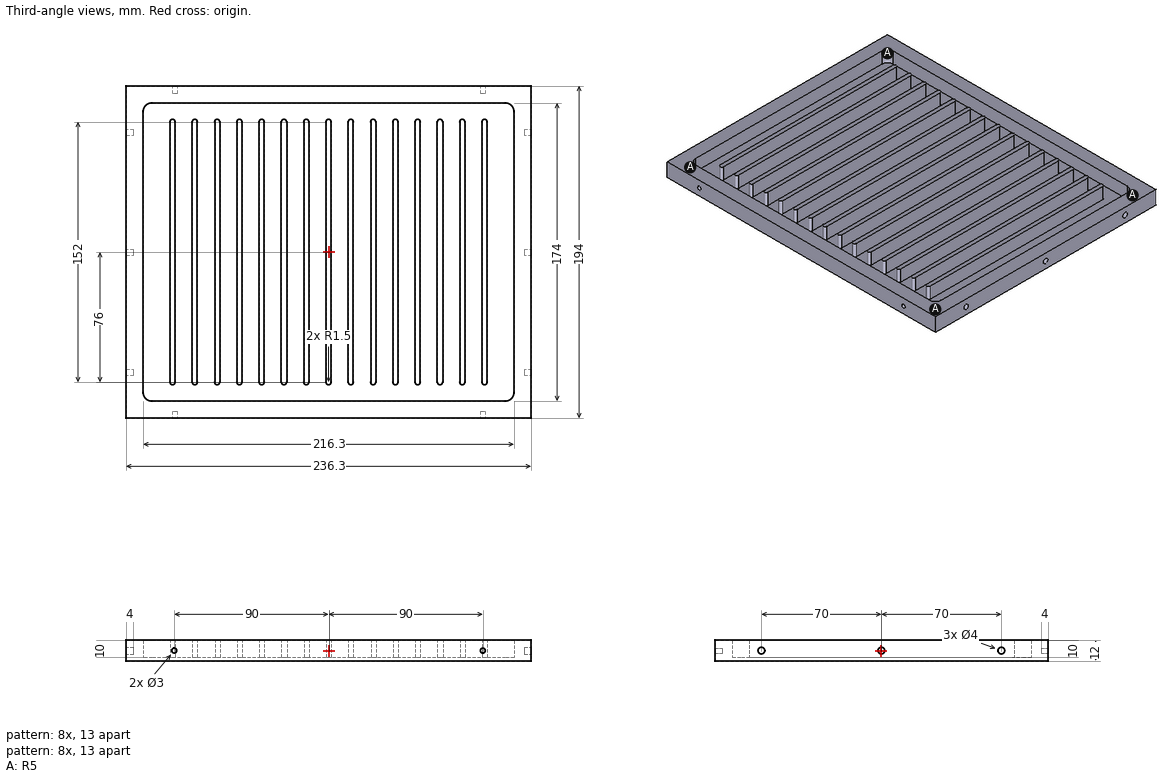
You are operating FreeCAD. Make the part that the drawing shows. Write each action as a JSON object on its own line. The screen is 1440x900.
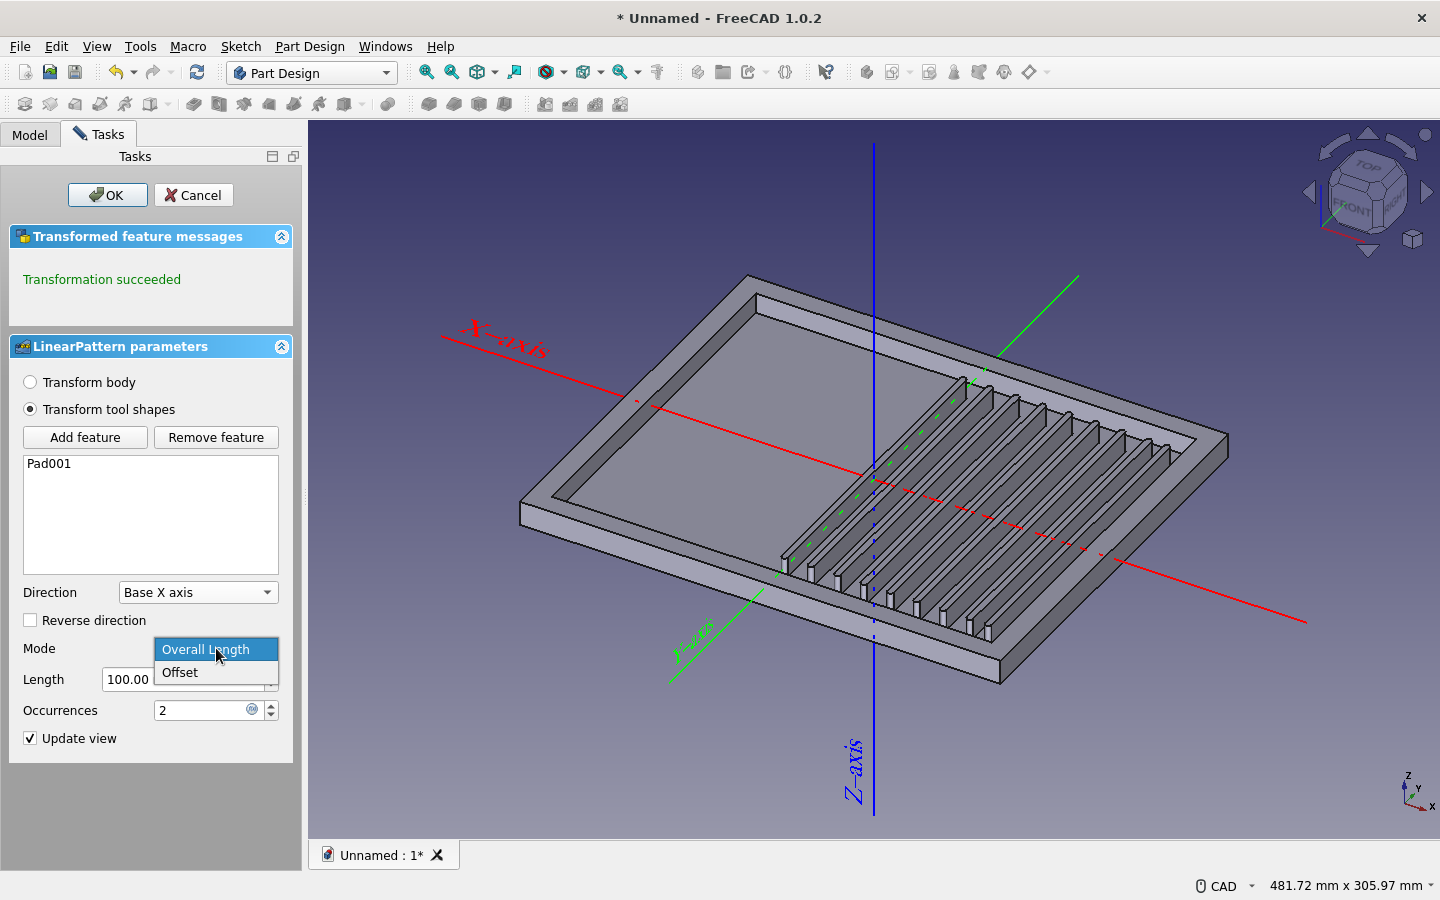
{"action": "left_click", "coordinate": [214, 672]}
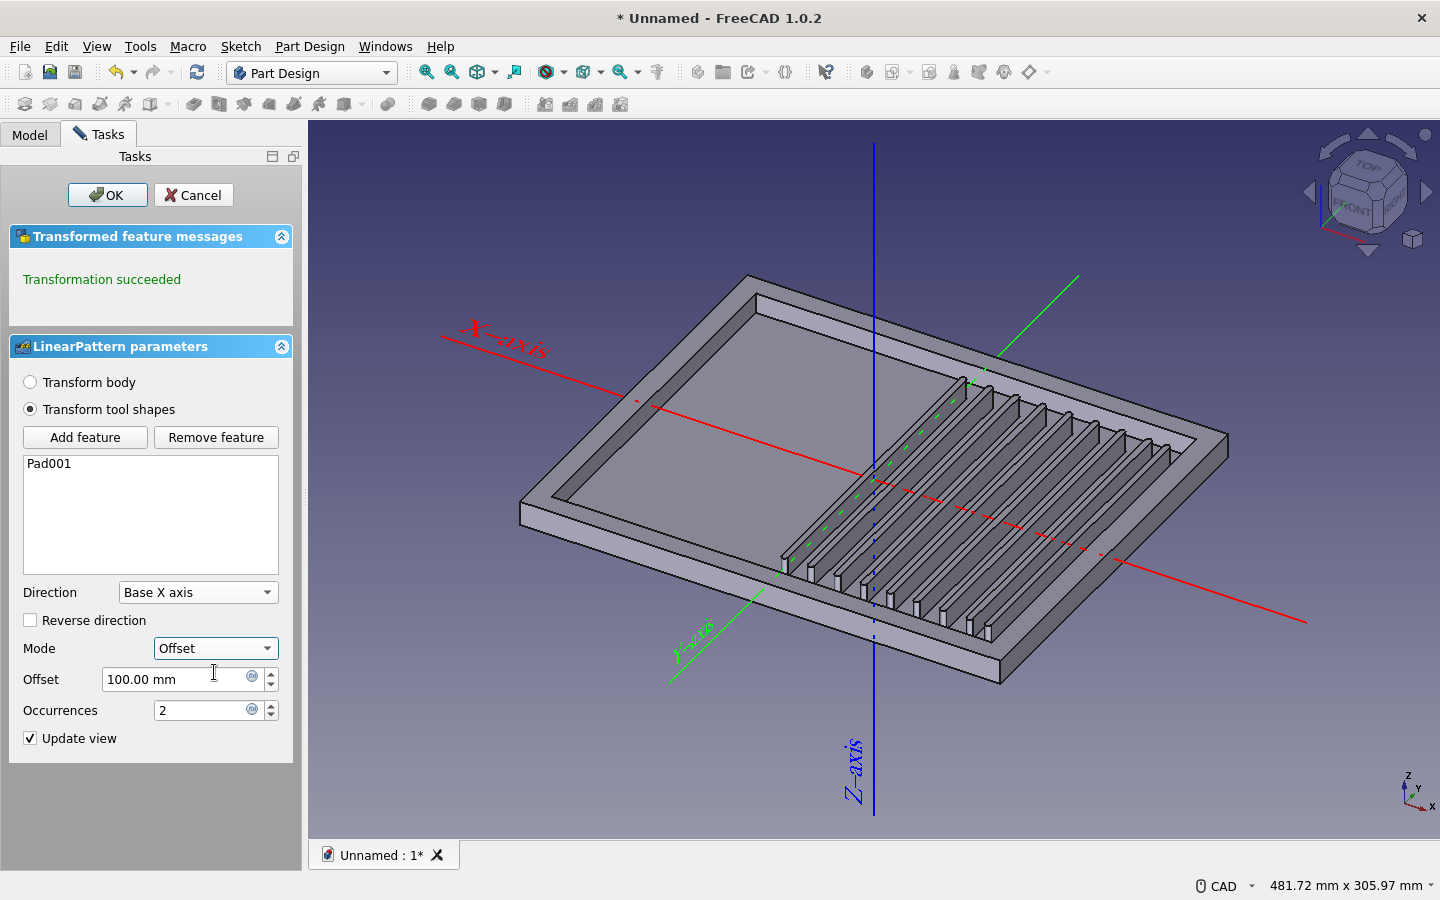
{"action": "triple_click", "coordinate": [184, 680]}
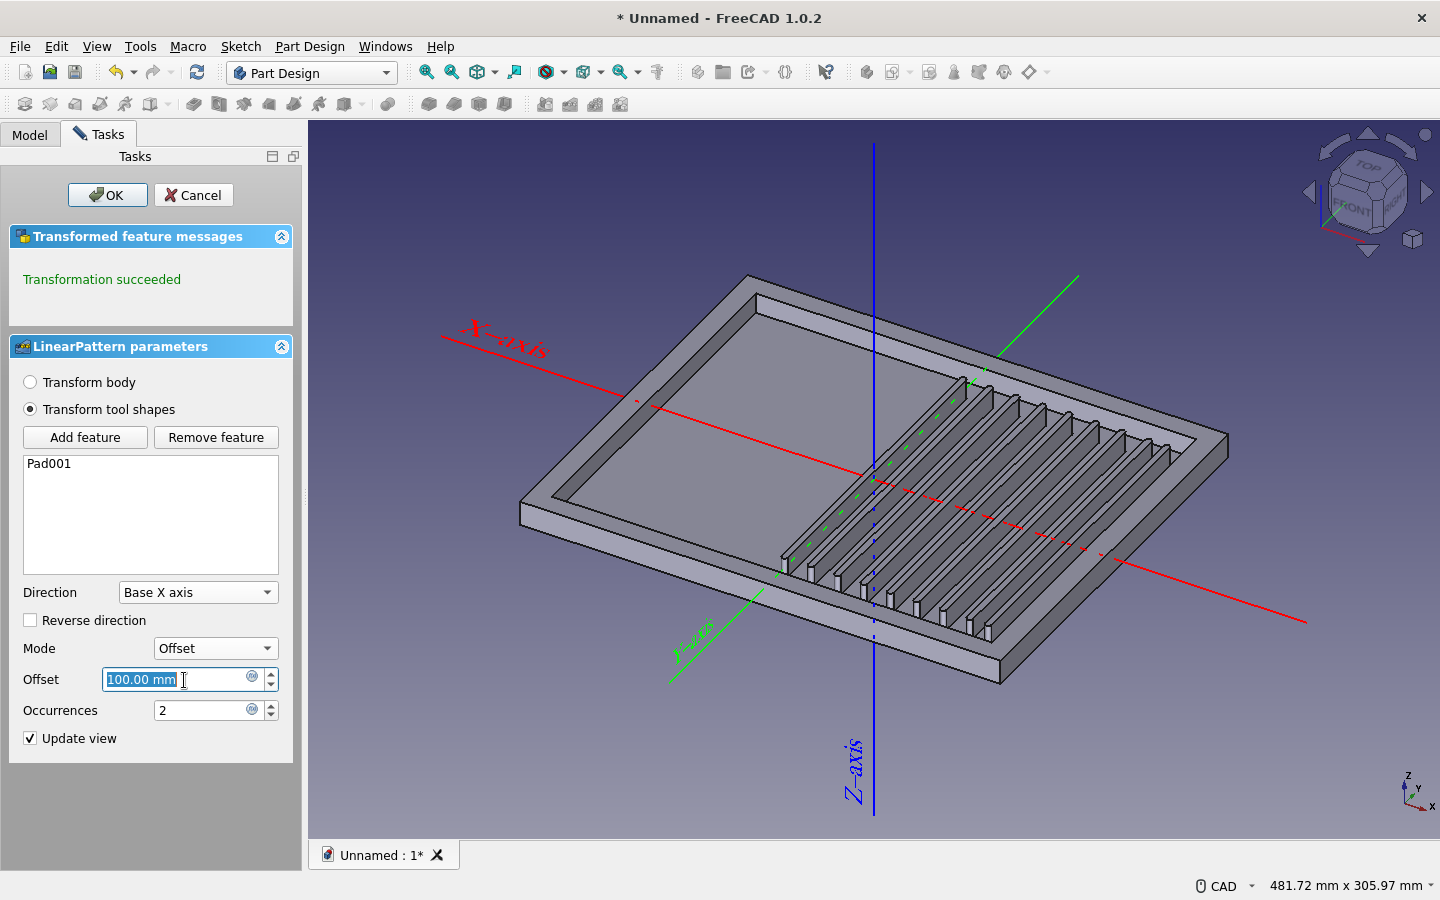
{"action": "type", "text": "13"}
{"action": "key", "text": "Tab"}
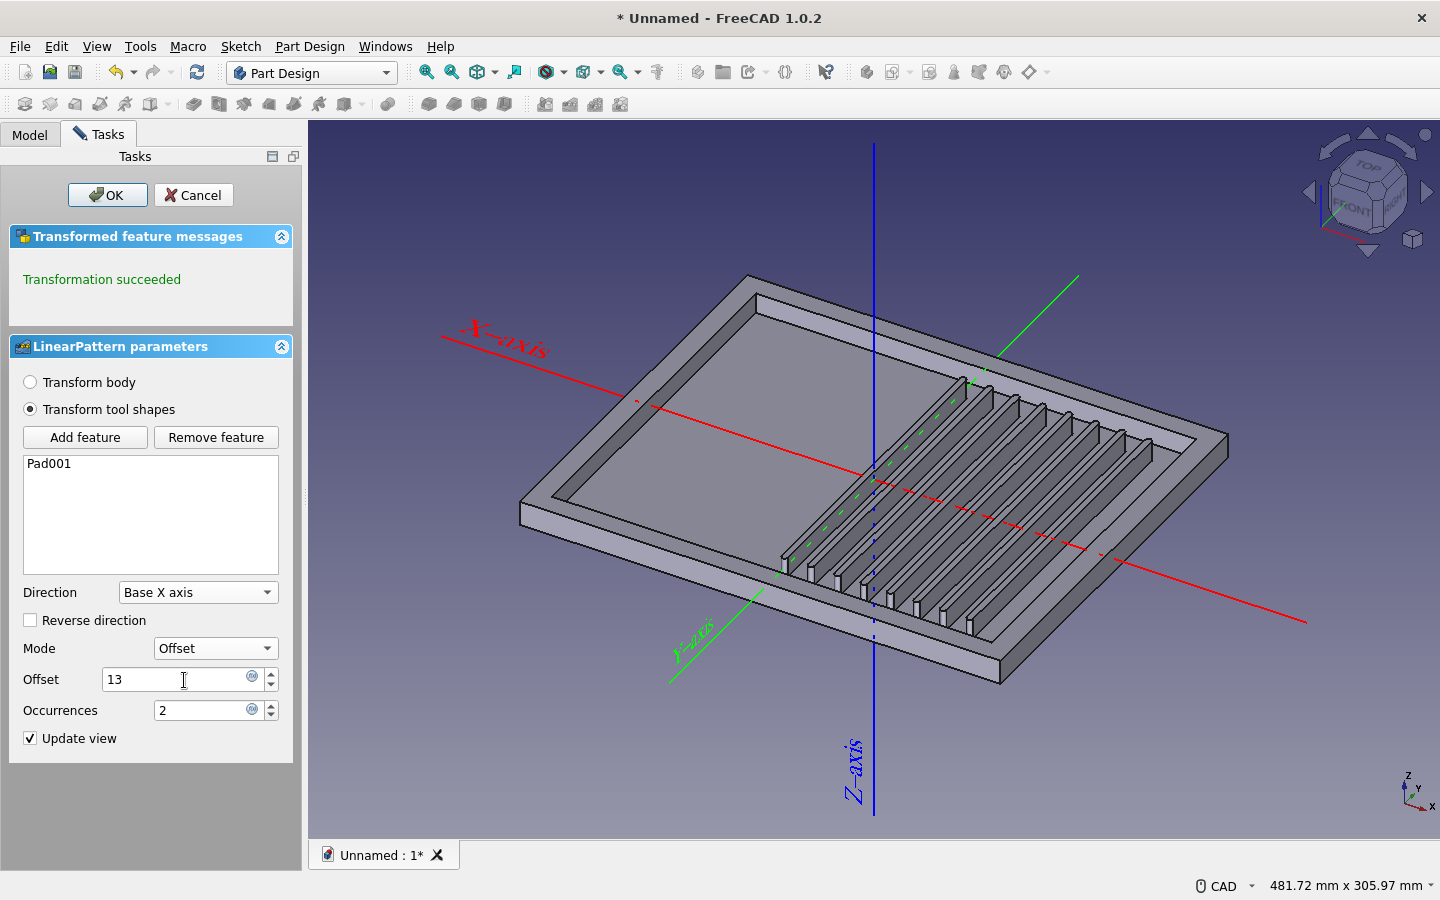
{"action": "triple_click", "coordinate": [210, 710]}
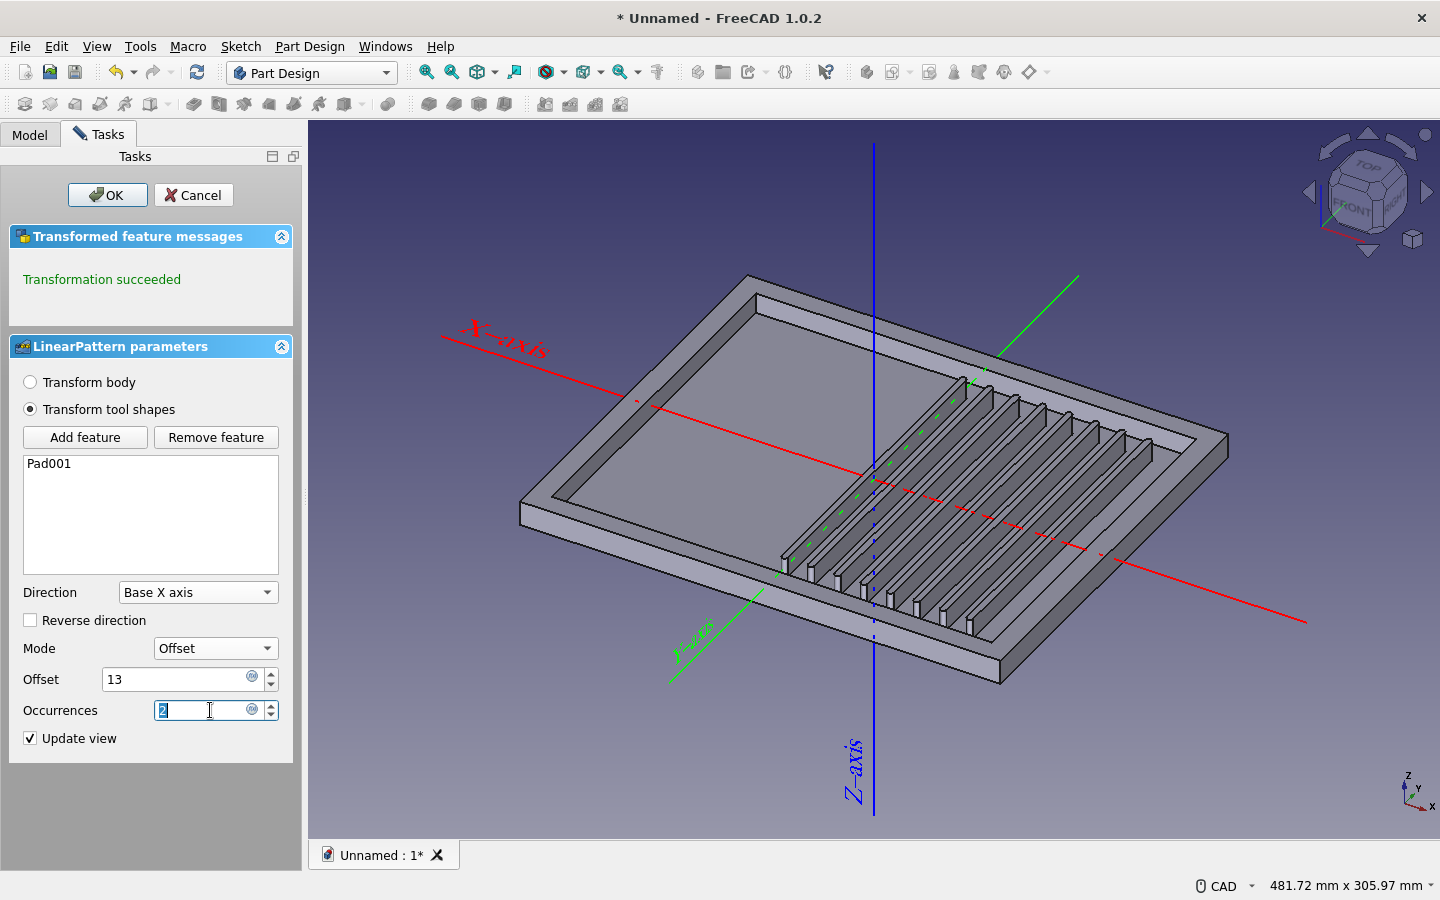
{"action": "type", "text": "8"}
{"action": "key", "text": "Tab"}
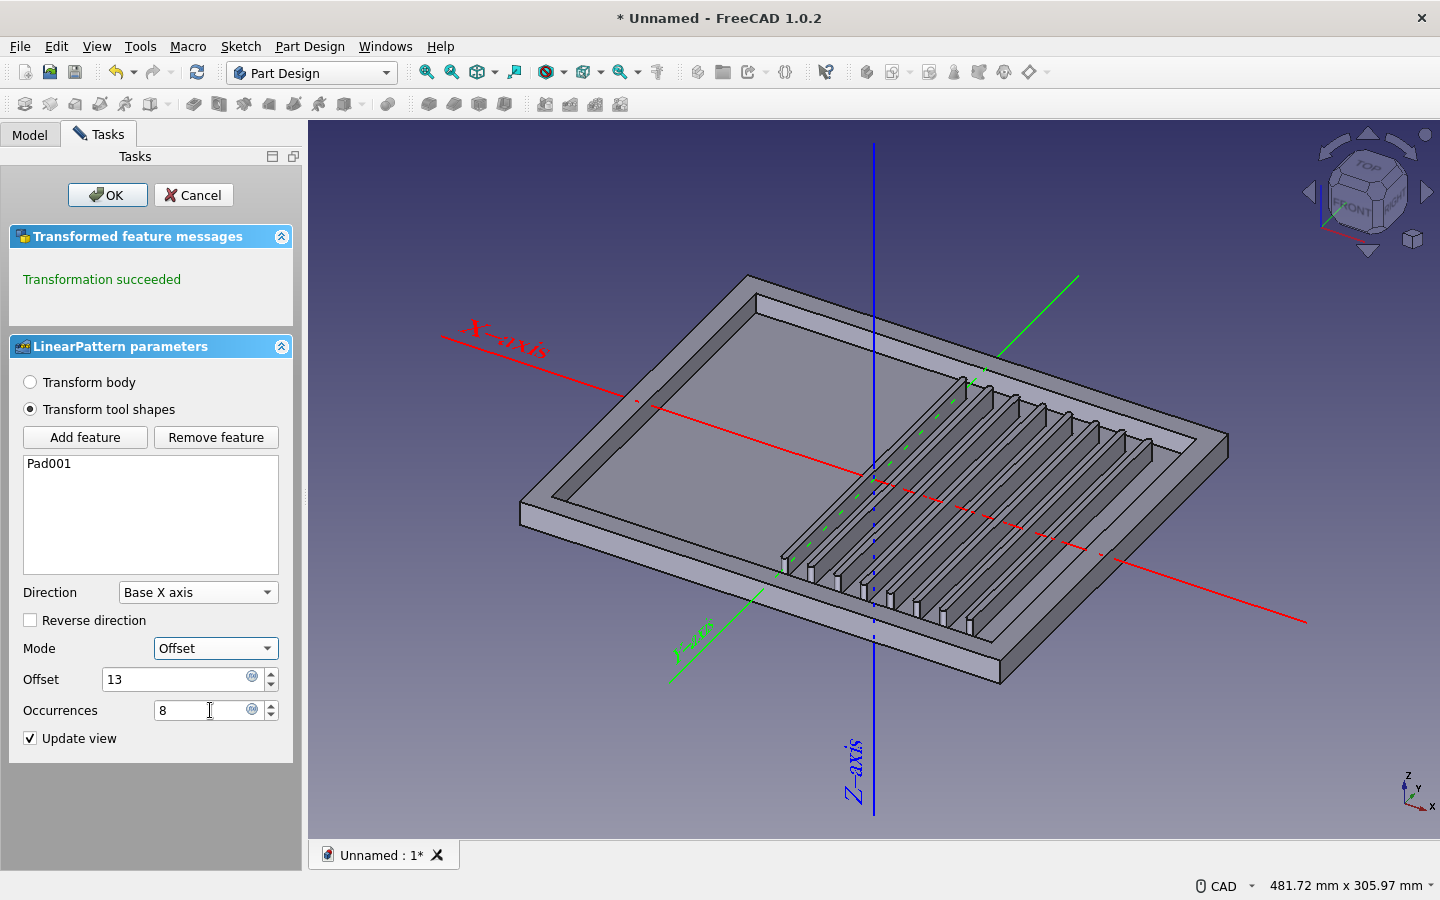
{"action": "left_click", "coordinate": [31, 620]}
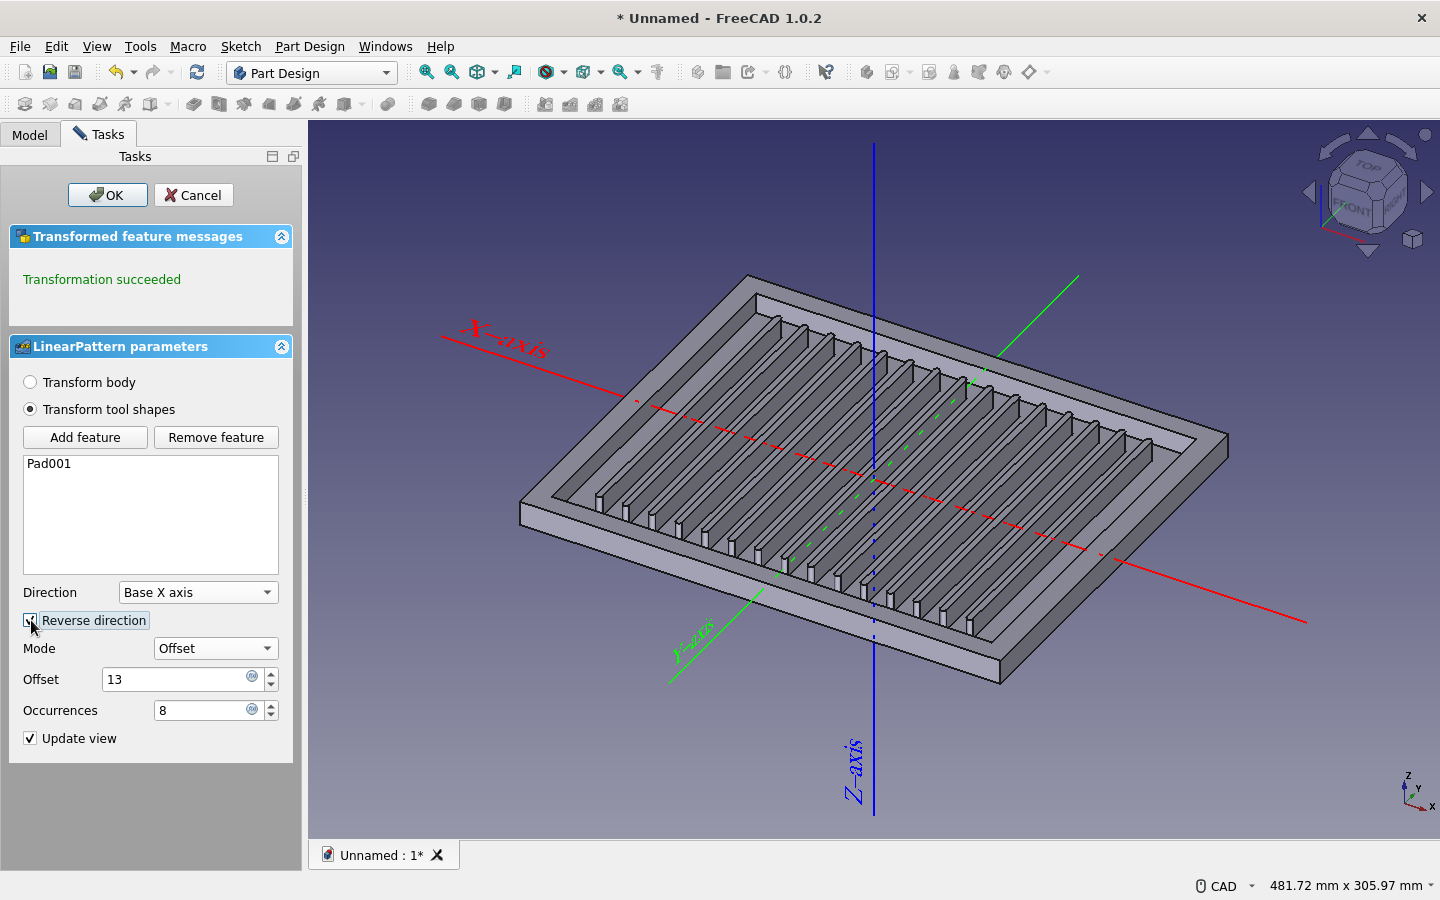
{"action": "left_click", "coordinate": [108, 195]}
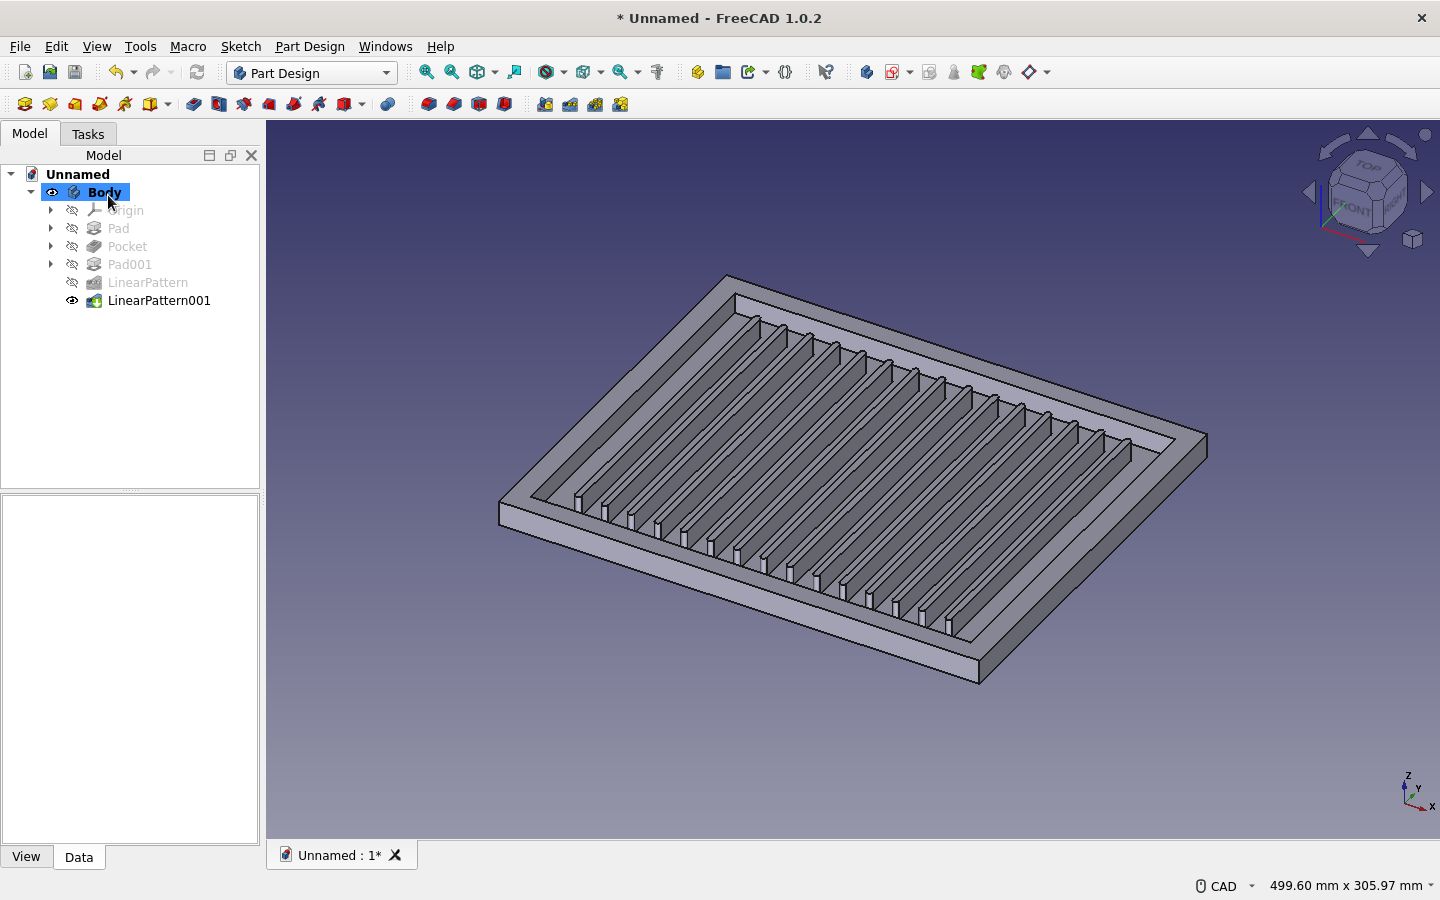
{"action": "key", "text": "4"}